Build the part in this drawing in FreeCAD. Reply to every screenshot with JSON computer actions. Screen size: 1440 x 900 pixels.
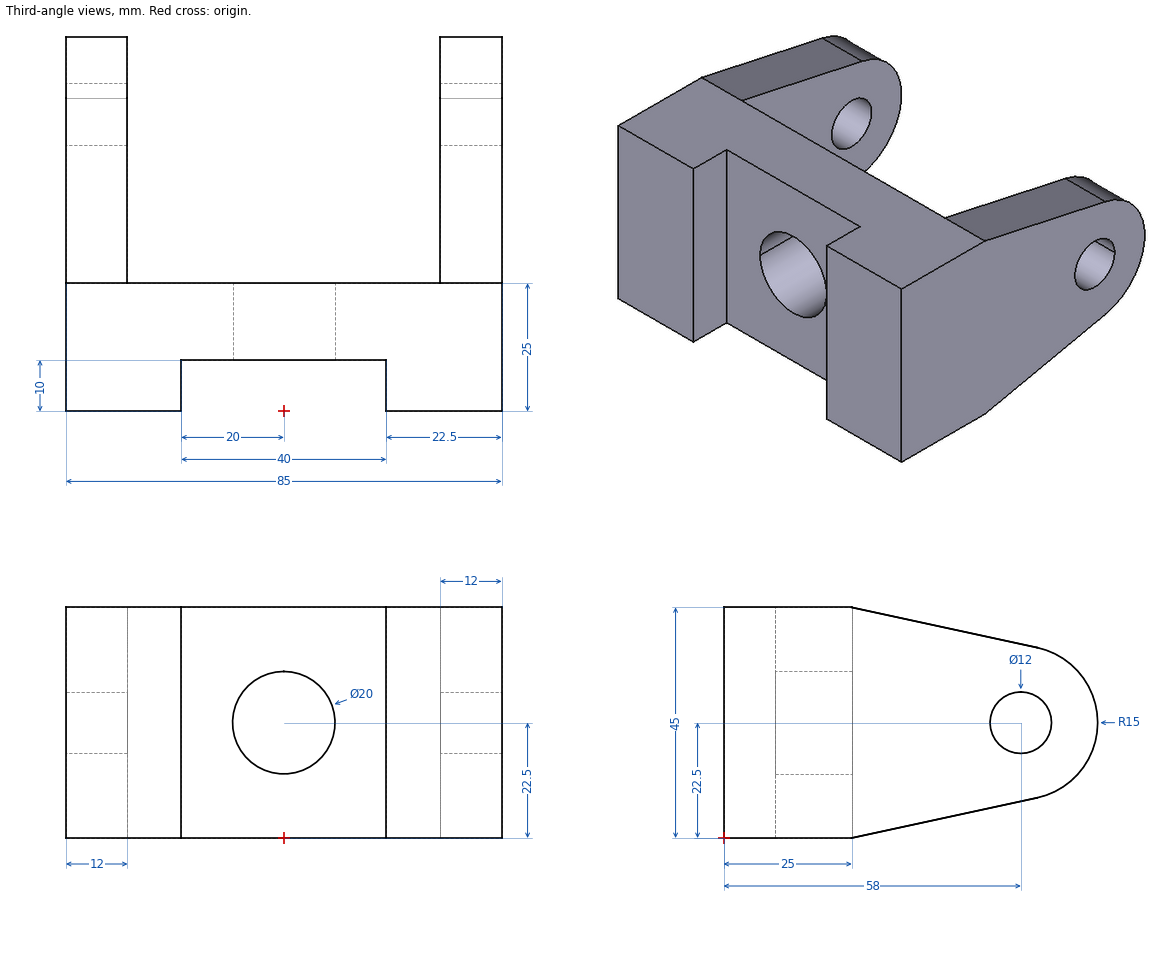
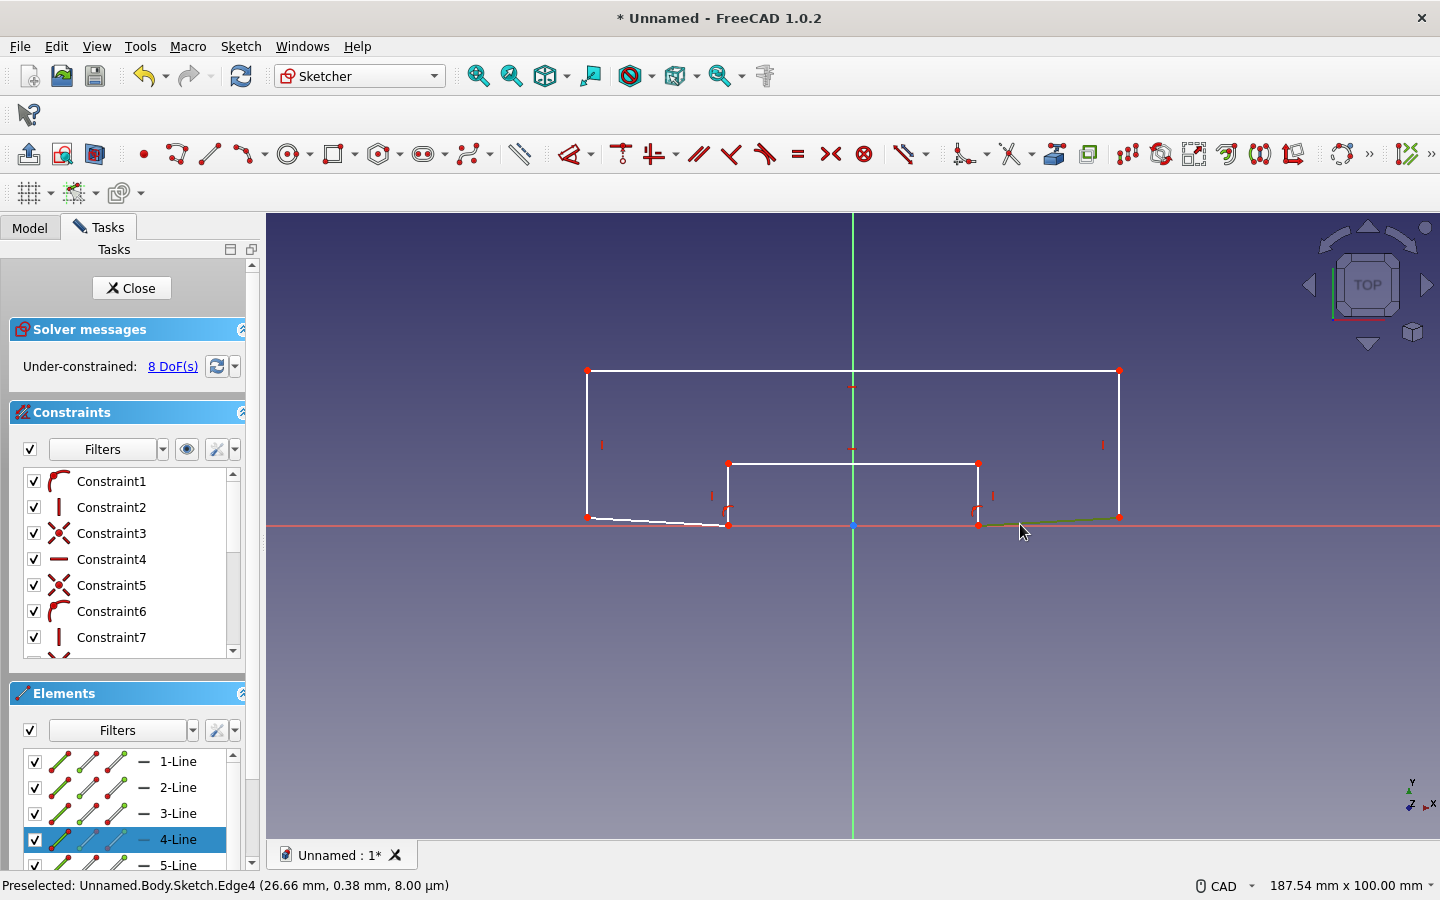
{"action": "key", "text": "h"}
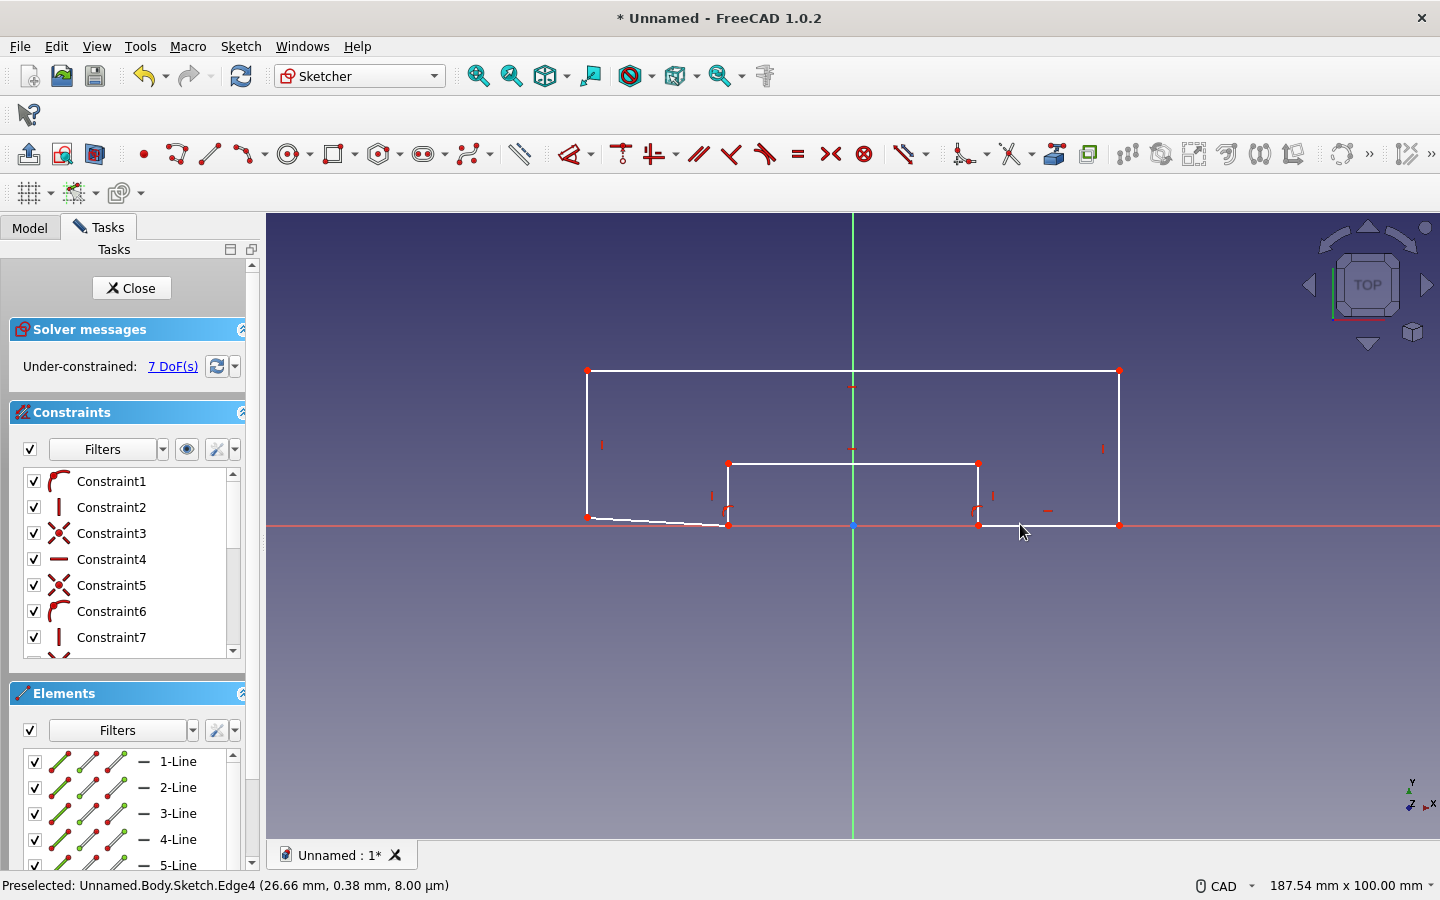
{"action": "left_click", "coordinate": [686, 524]}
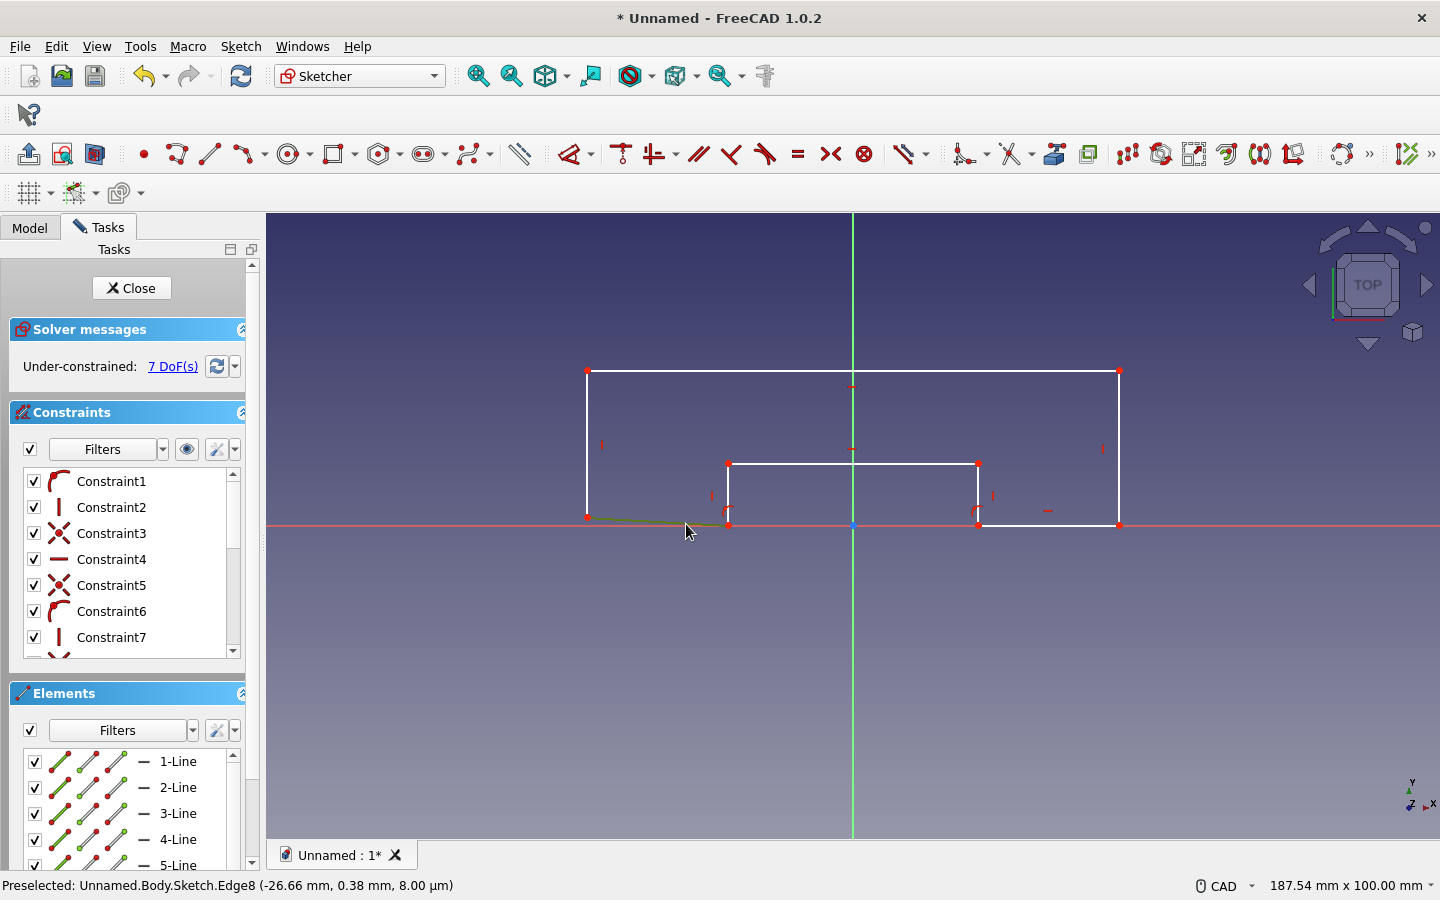
{"action": "key", "text": "h"}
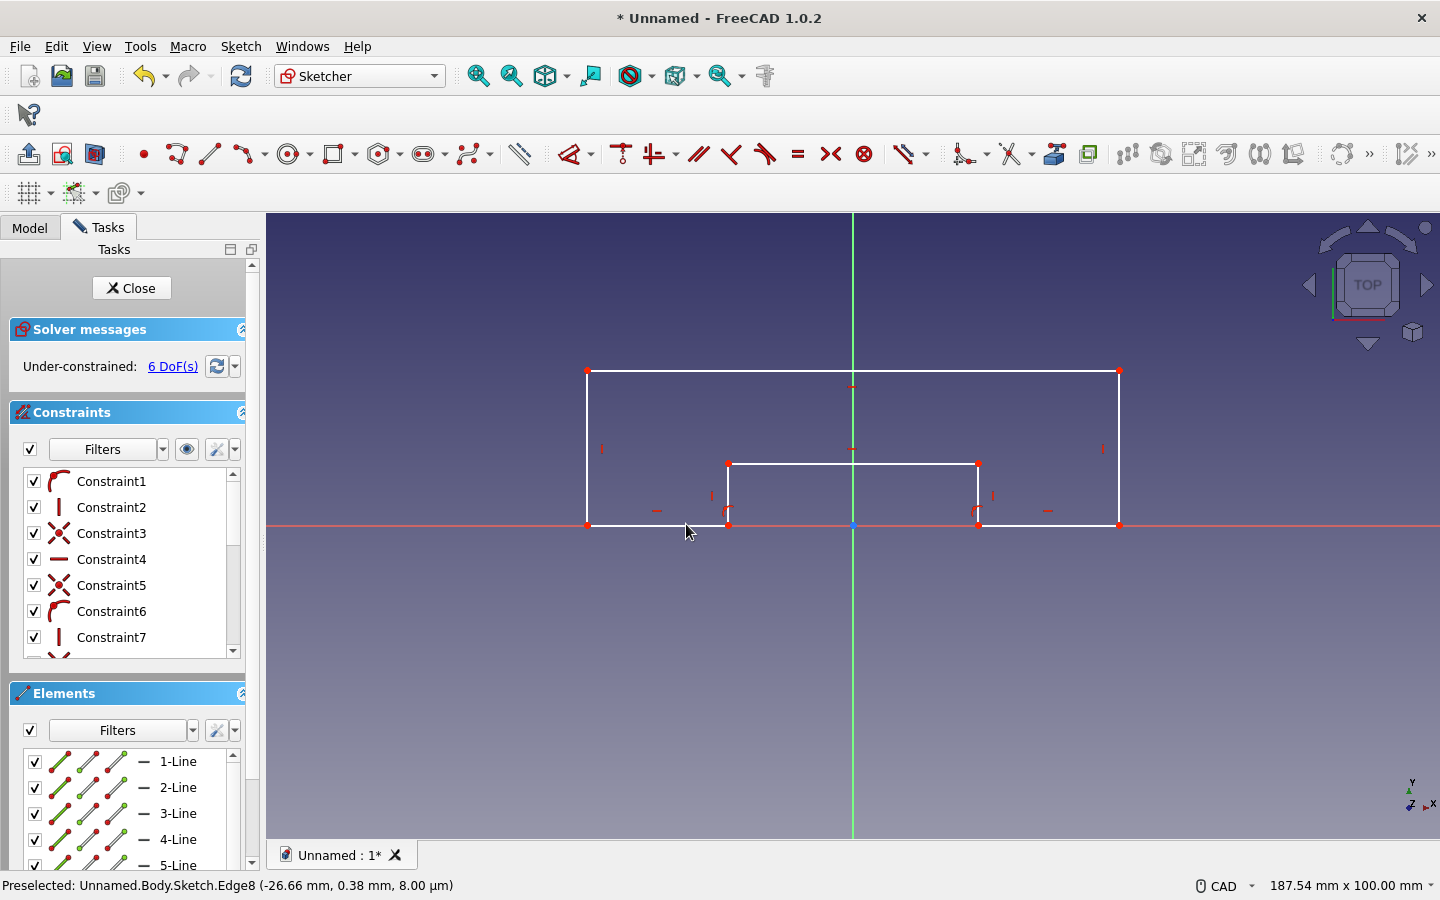
{"action": "left_click", "coordinate": [568, 154]}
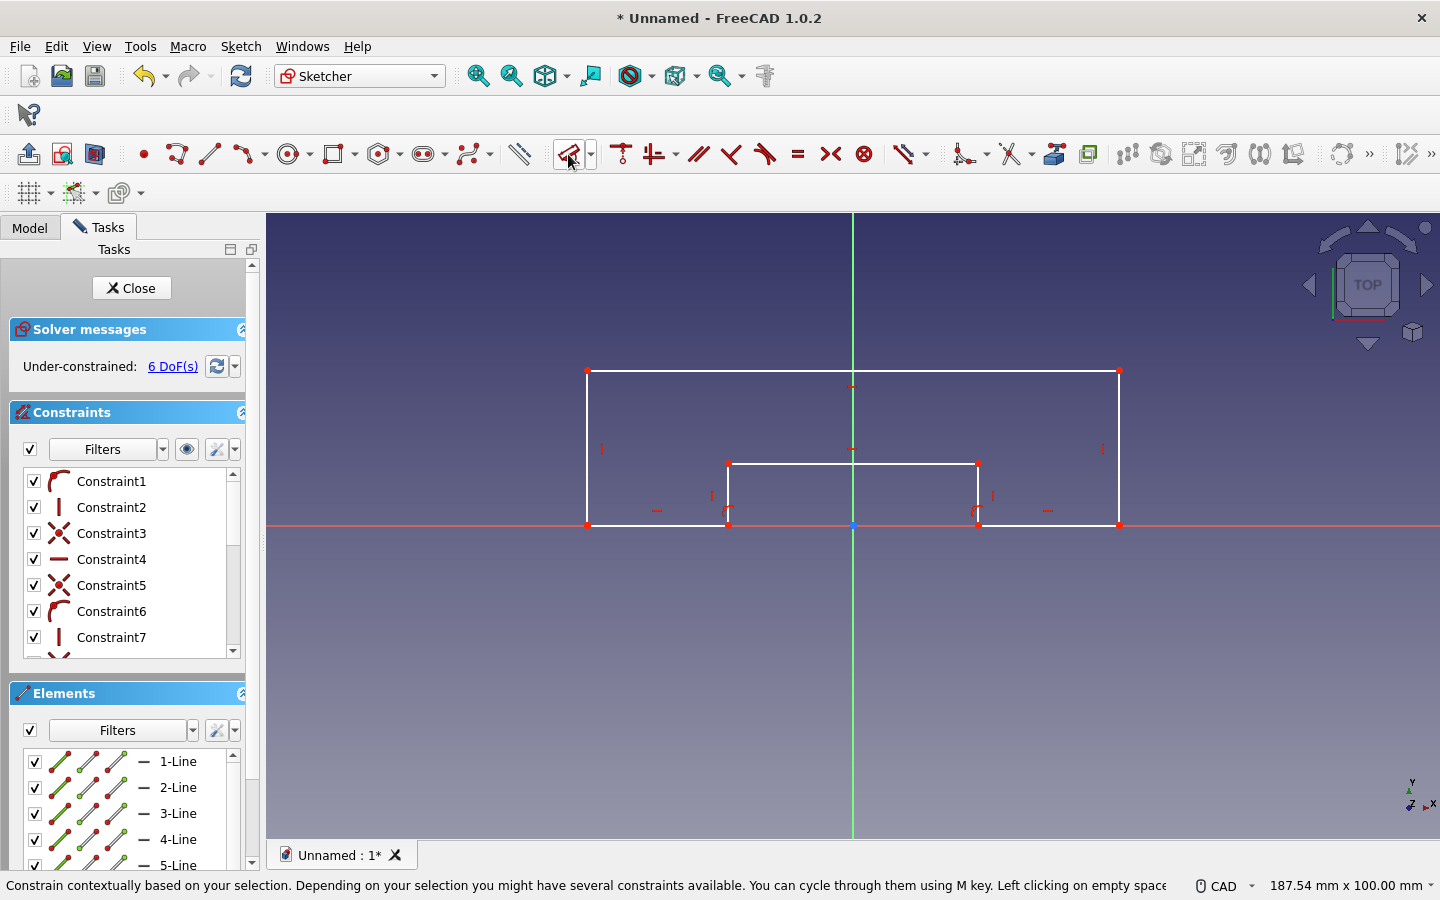
{"action": "left_click", "coordinate": [728, 507]}
{"action": "left_click", "coordinate": [694, 495]}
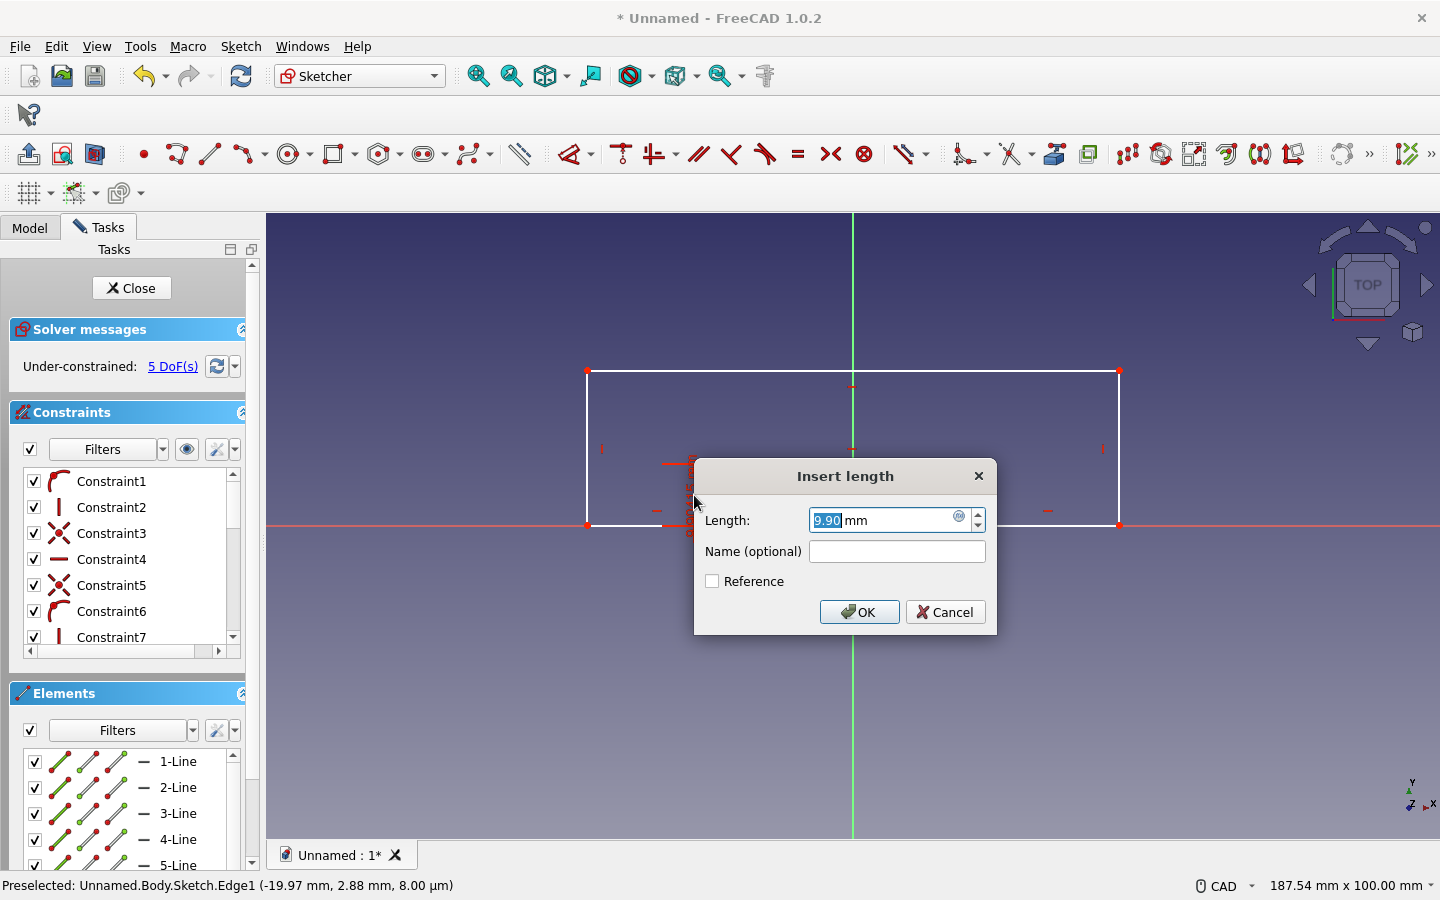
{"action": "type", "text": "10"}
{"action": "key", "text": "Return"}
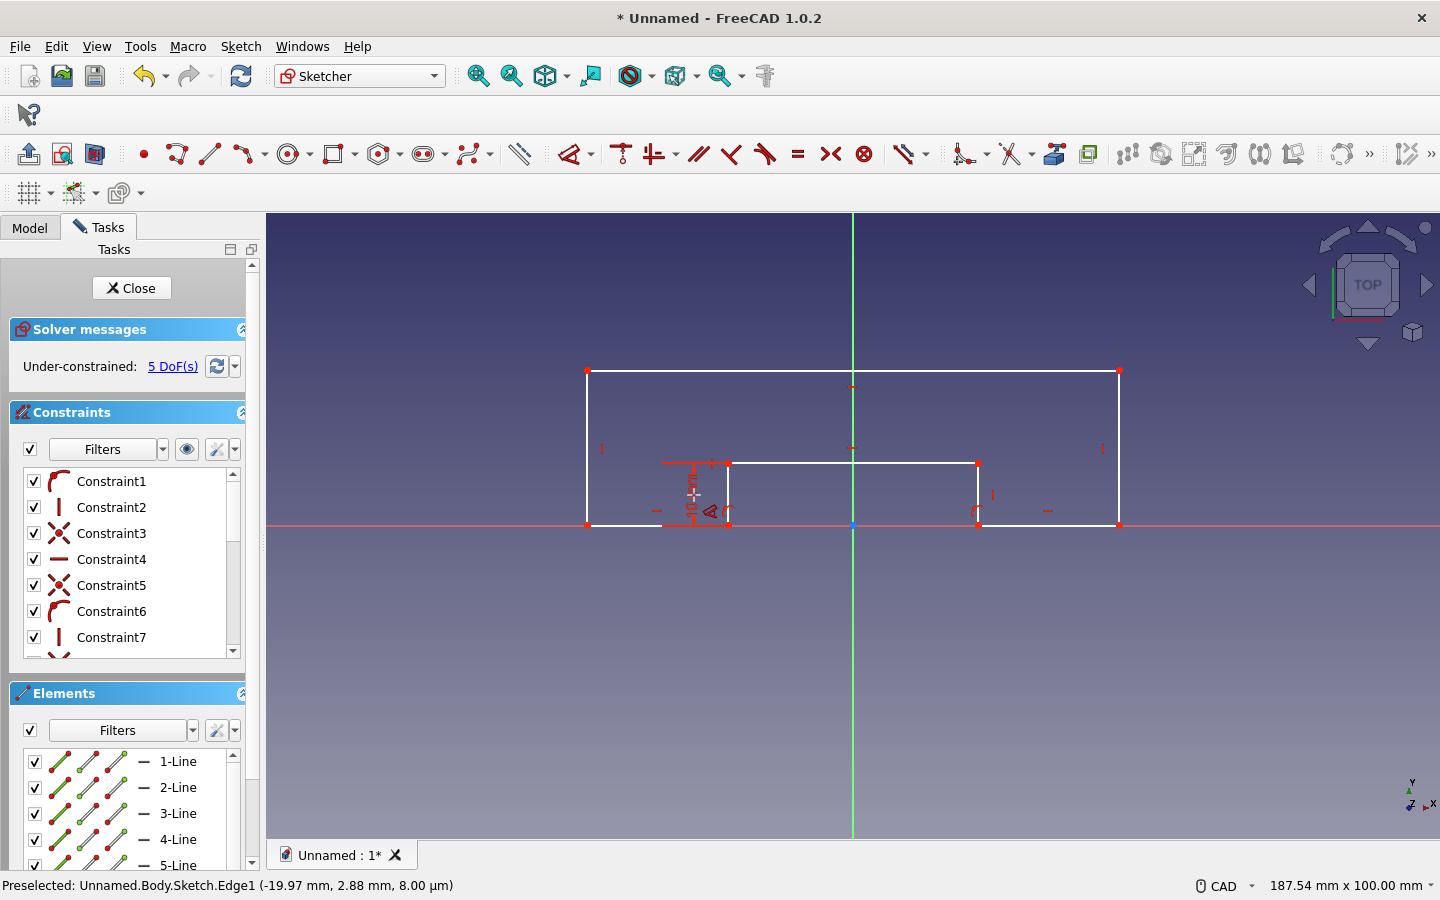
{"action": "left_click", "coordinate": [803, 463]}
{"action": "left_click", "coordinate": [795, 497]}